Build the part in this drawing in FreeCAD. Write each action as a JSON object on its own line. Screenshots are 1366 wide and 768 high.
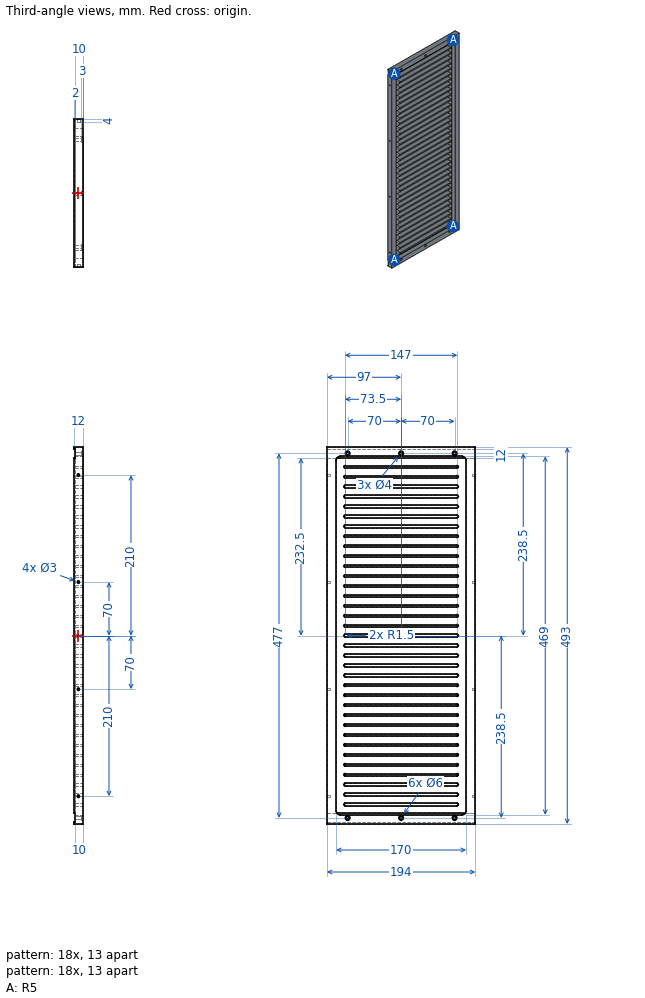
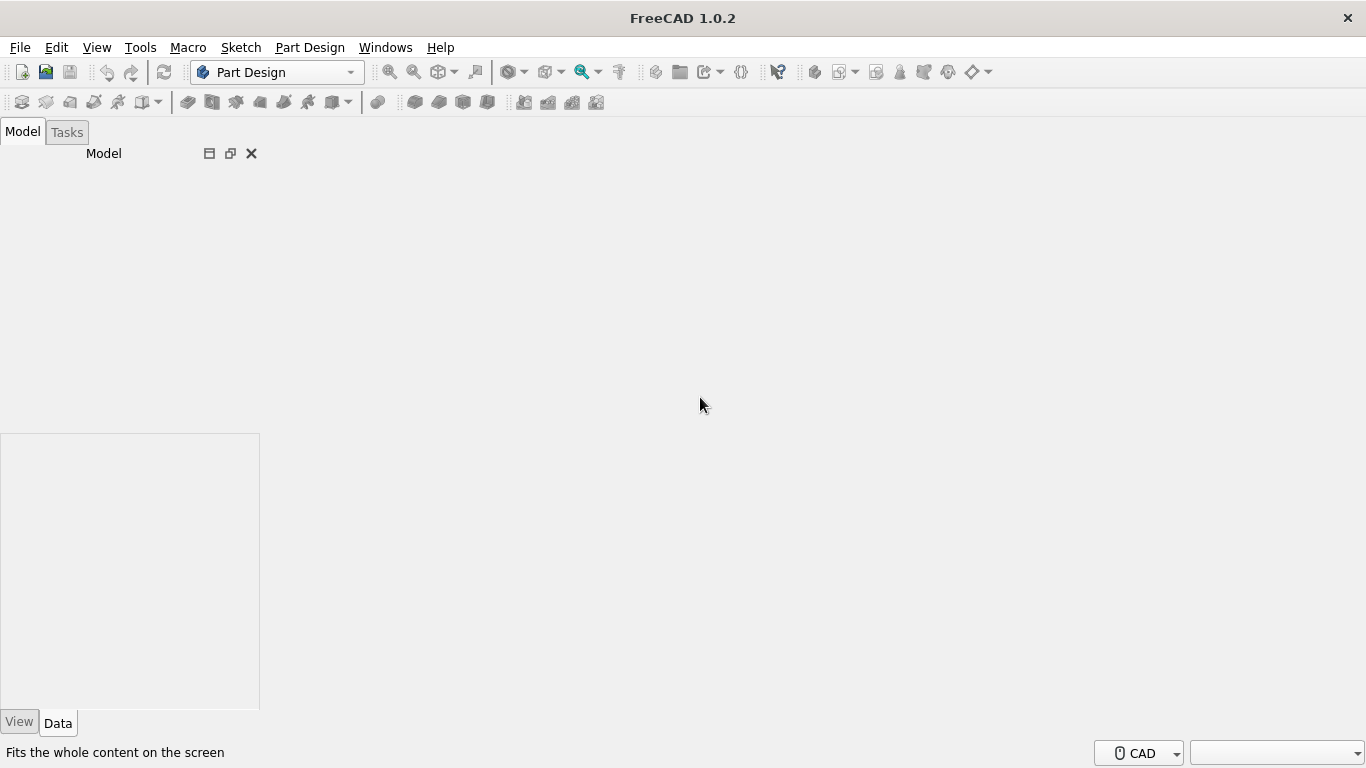
{"action": "left_click", "coordinate": [22, 72]}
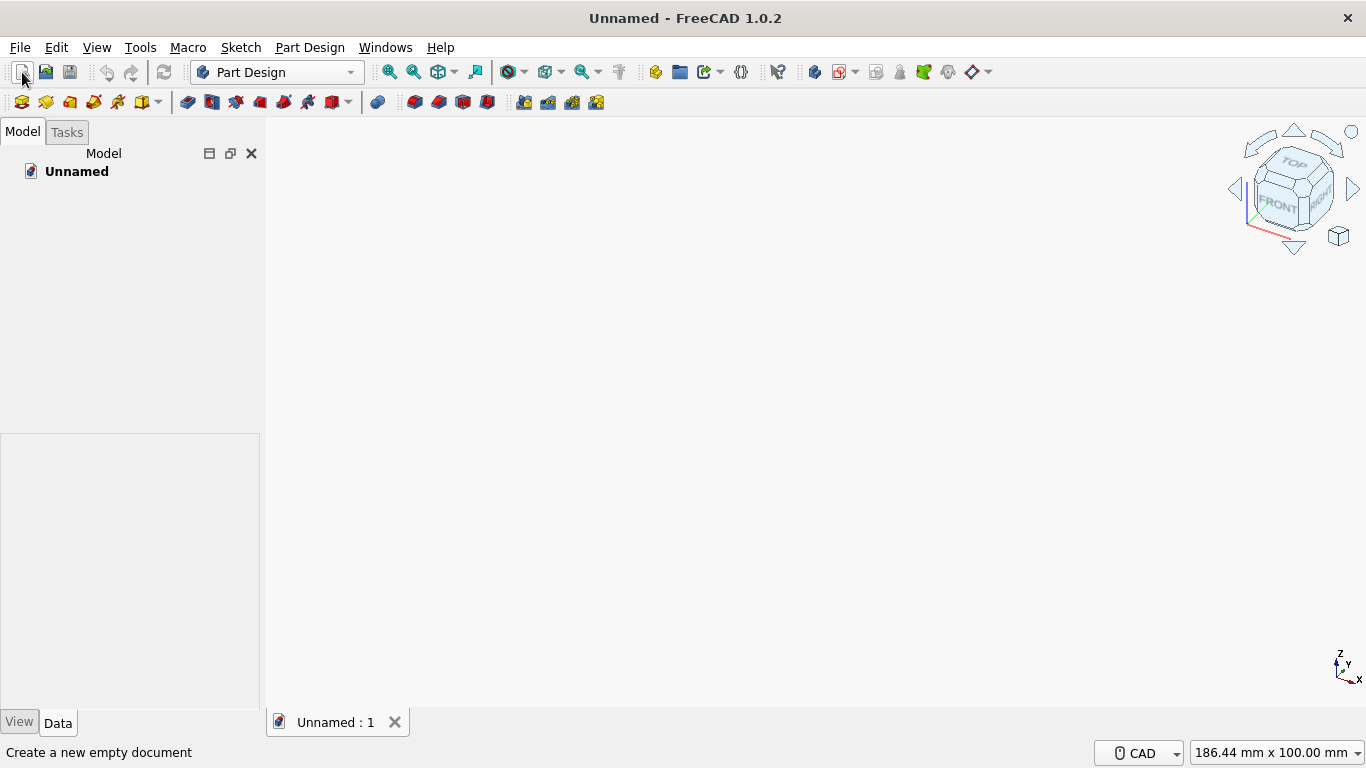
{"action": "left_click", "coordinate": [840, 72]}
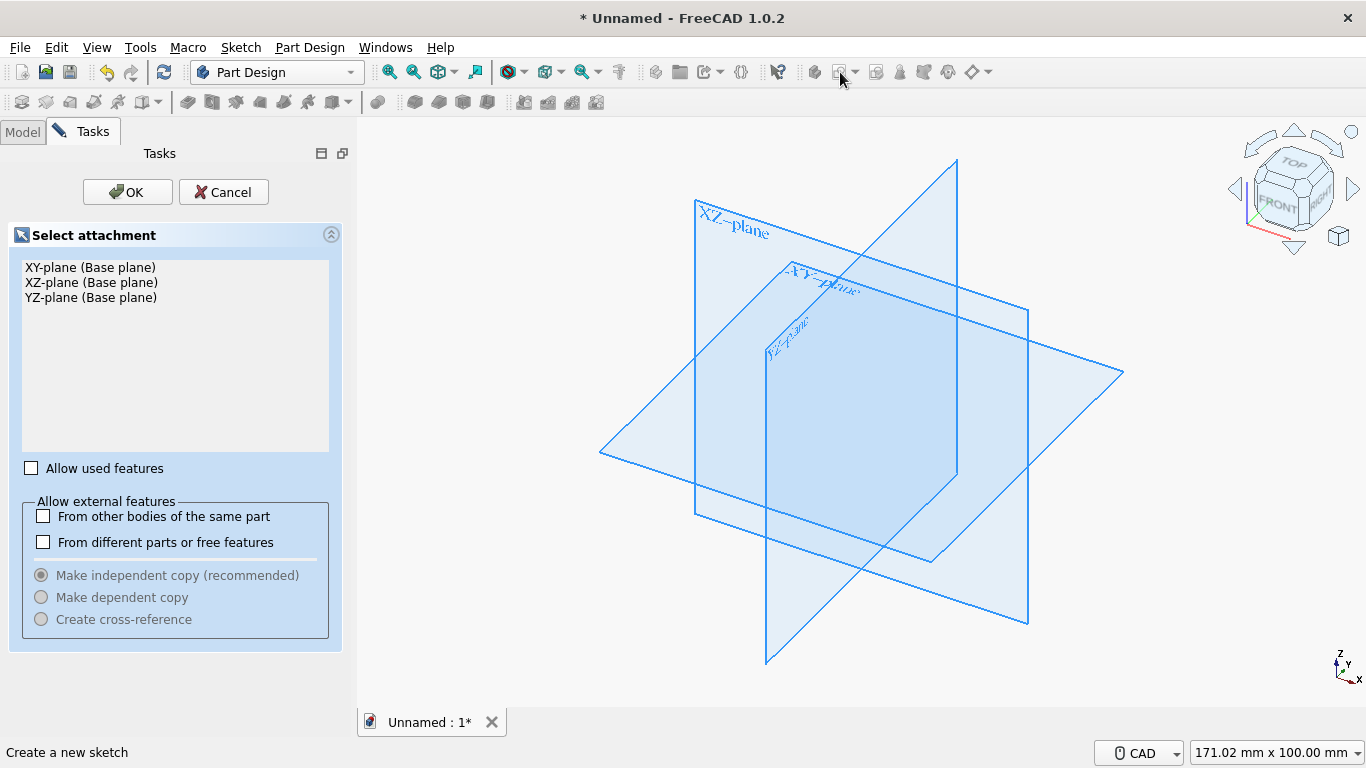
{"action": "left_click", "coordinate": [82, 298]}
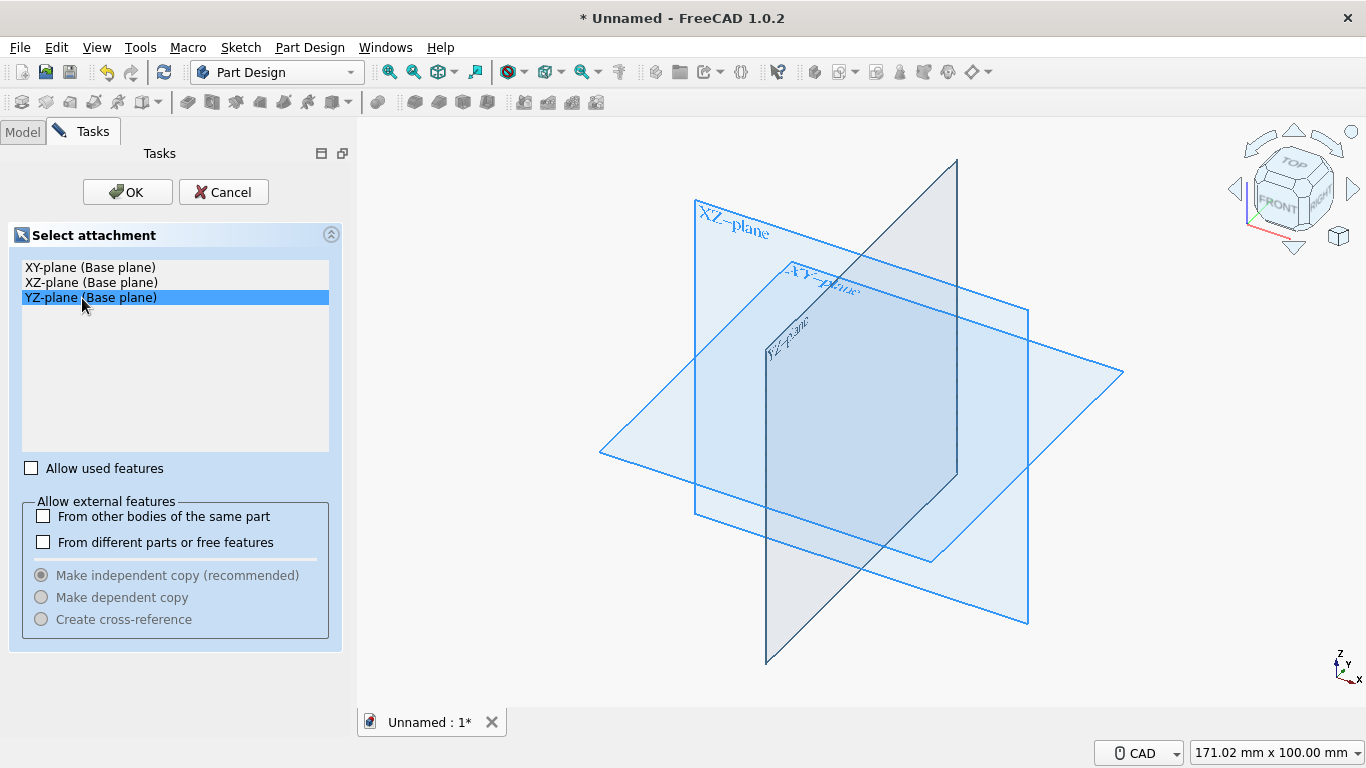
{"action": "left_click", "coordinate": [128, 192]}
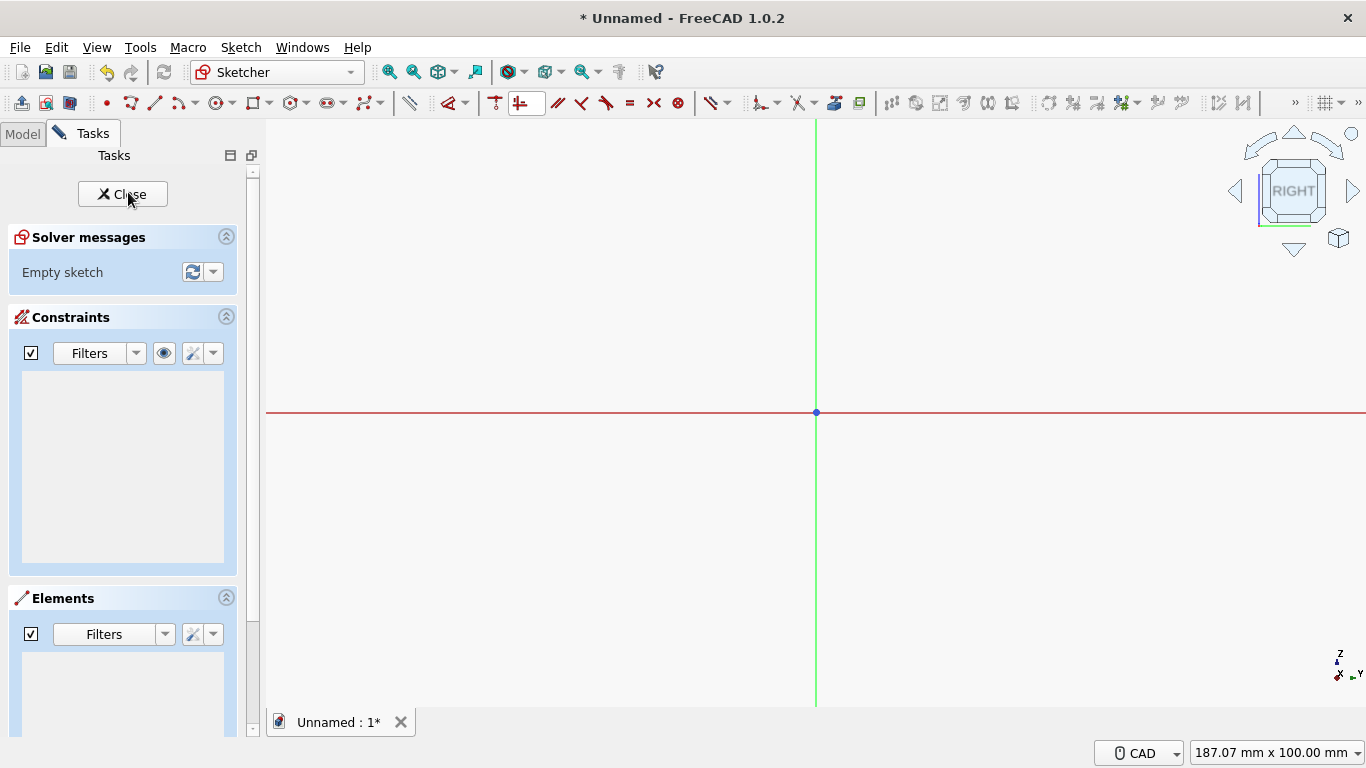
{"action": "scroll", "coordinate": [737, 413], "scroll_direction": "down", "scroll_amount": 10}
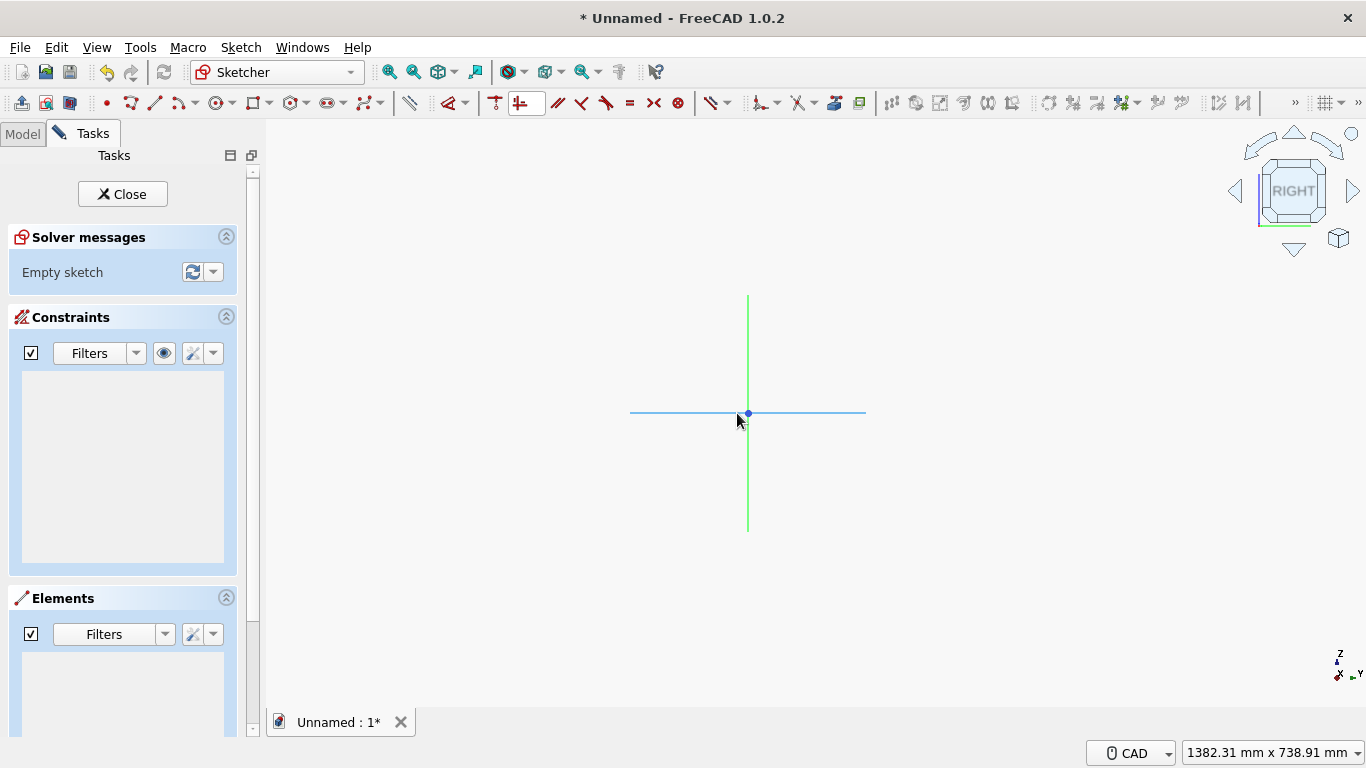
{"action": "left_click", "coordinate": [272, 104]}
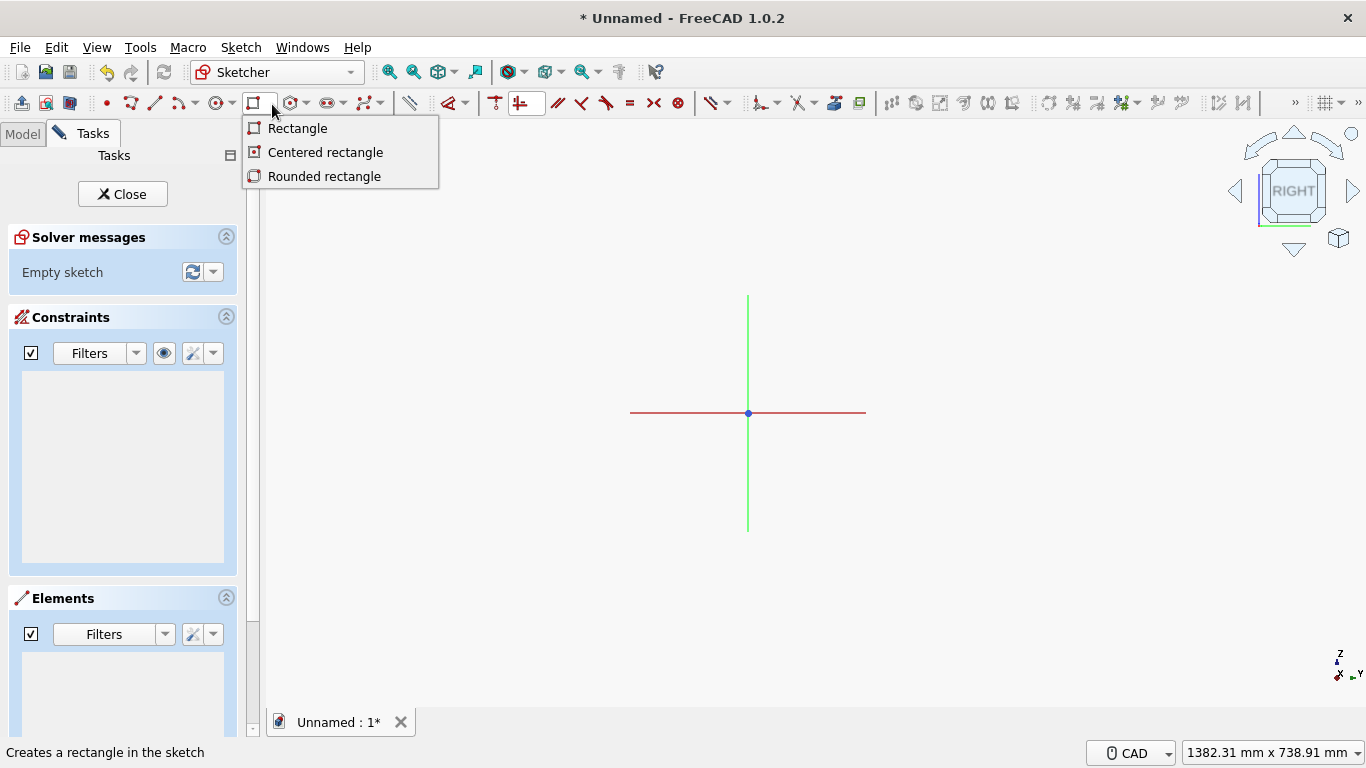
{"action": "left_click", "coordinate": [340, 152]}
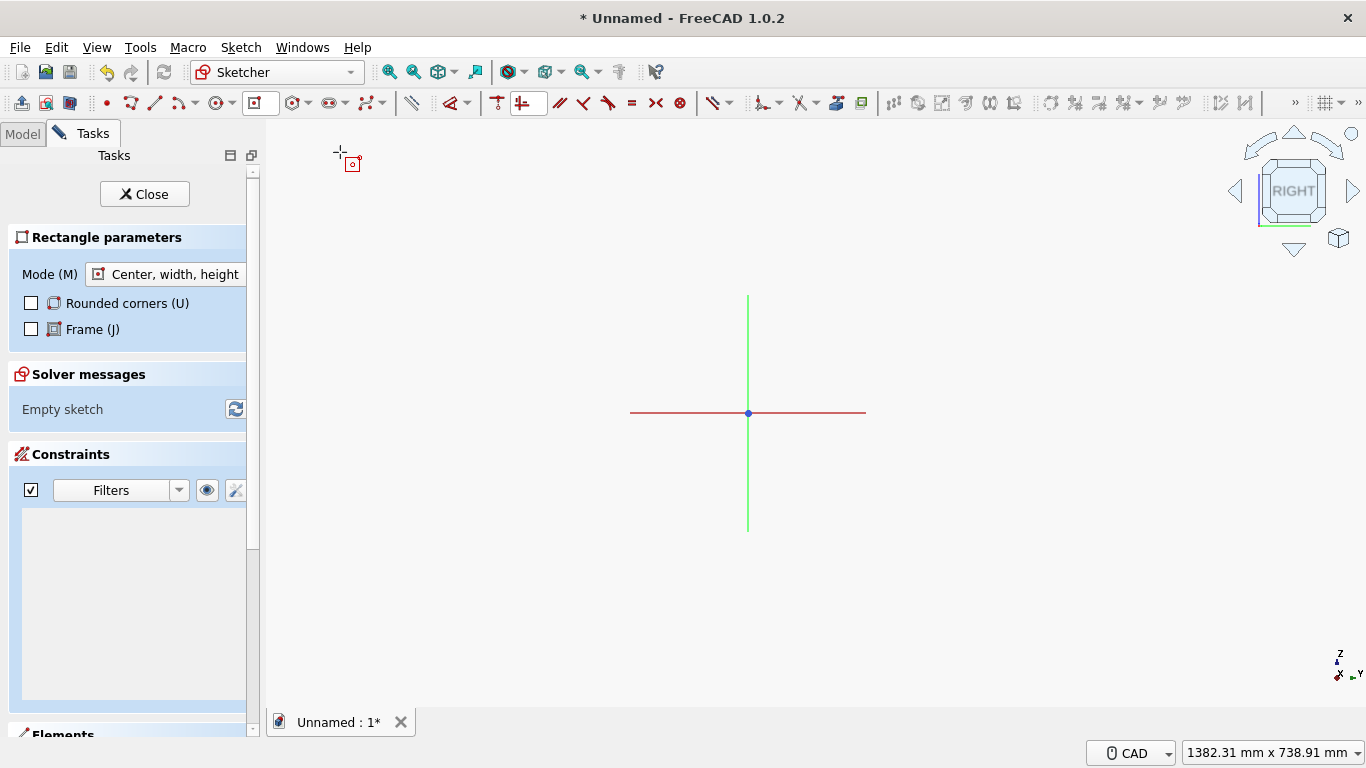
{"action": "left_click", "coordinate": [748, 413]}
{"action": "mouse_move", "coordinate": [825, 217]}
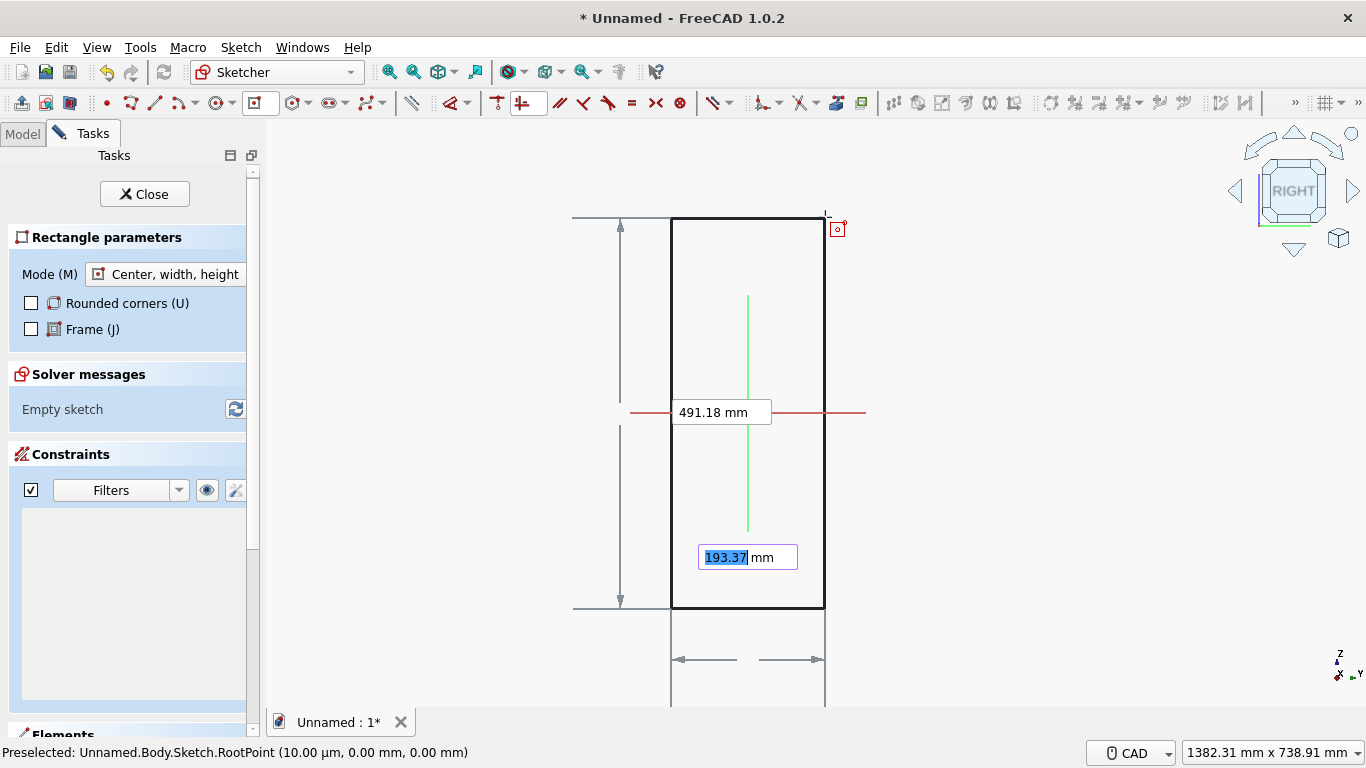
{"action": "type", "text": "194"}
{"action": "key", "text": "Tab"}
{"action": "type", "text": "493"}
{"action": "key", "text": "Return"}
{"action": "key", "text": "Escape"}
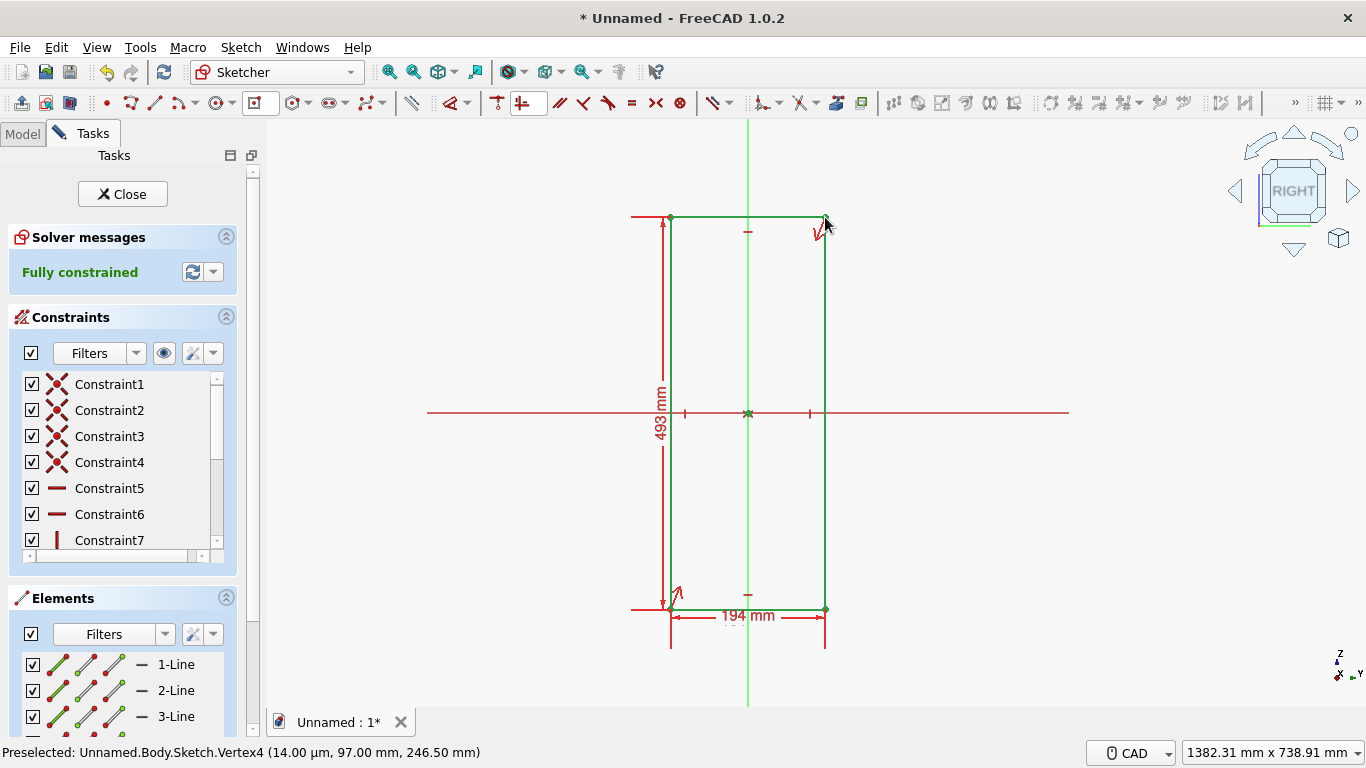
{"action": "left_click", "coordinate": [123, 194]}